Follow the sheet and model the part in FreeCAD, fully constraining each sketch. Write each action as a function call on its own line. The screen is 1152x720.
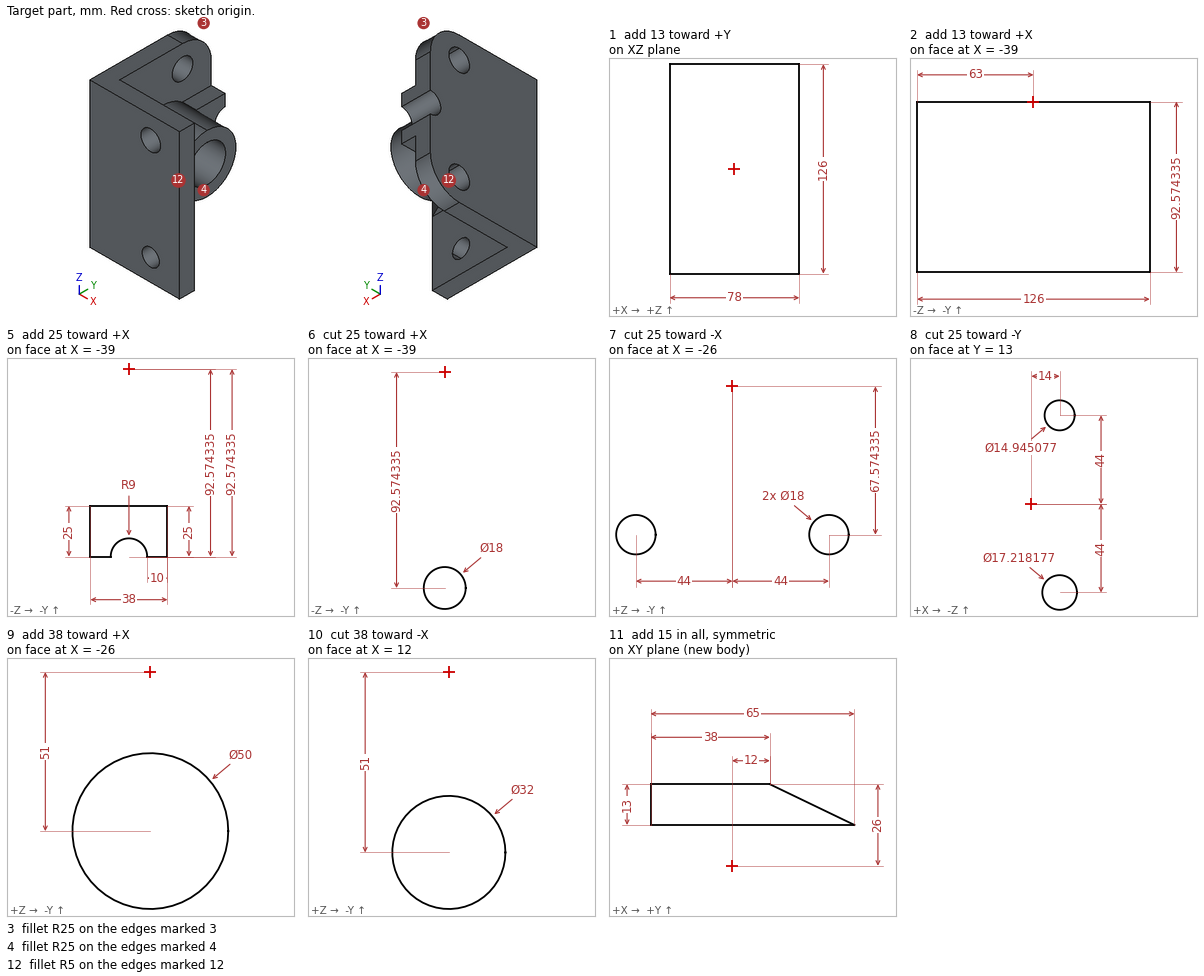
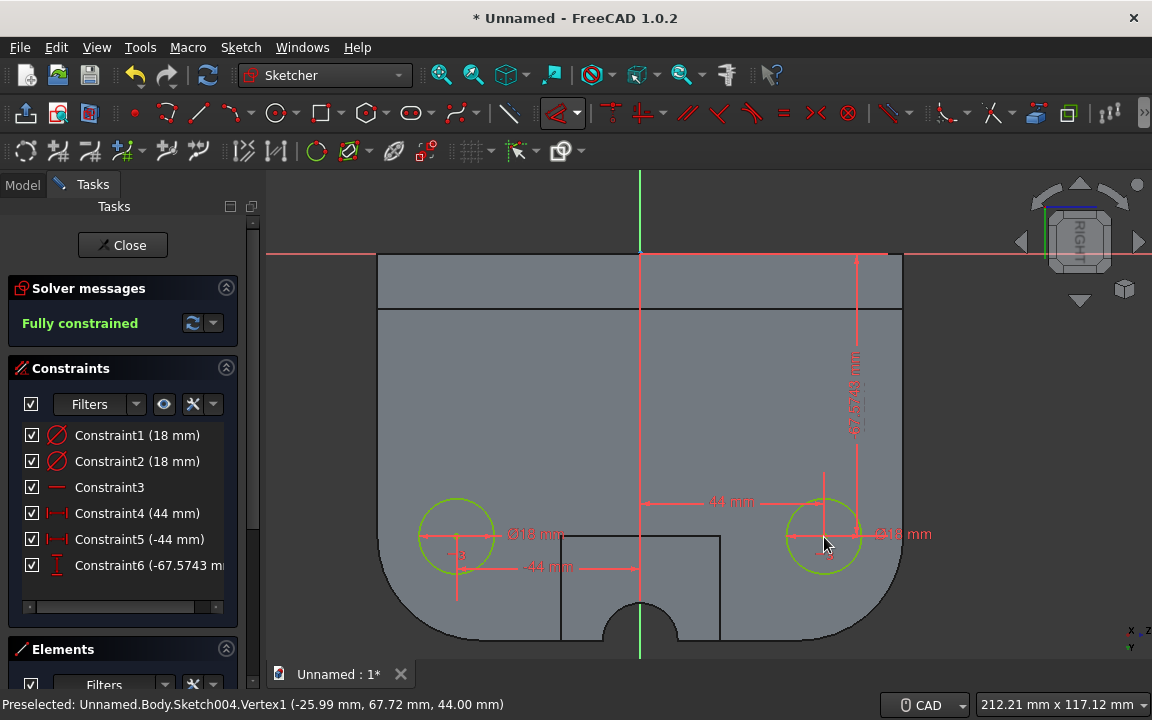
click(123, 245)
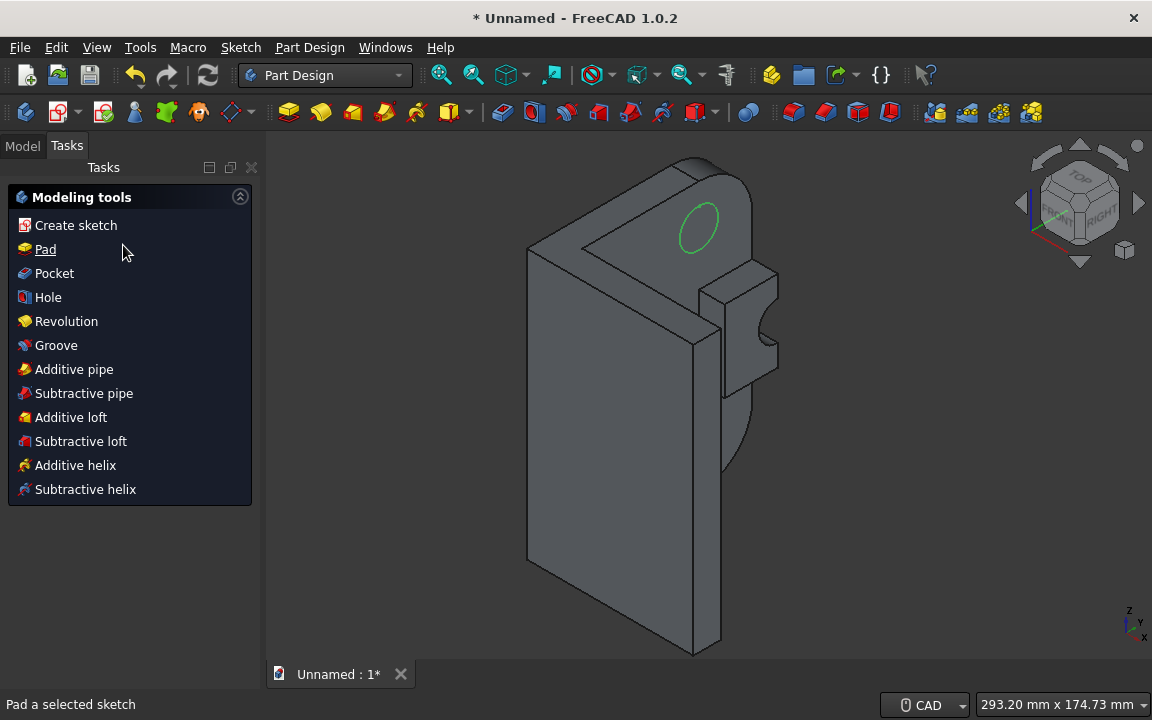
click(504, 112)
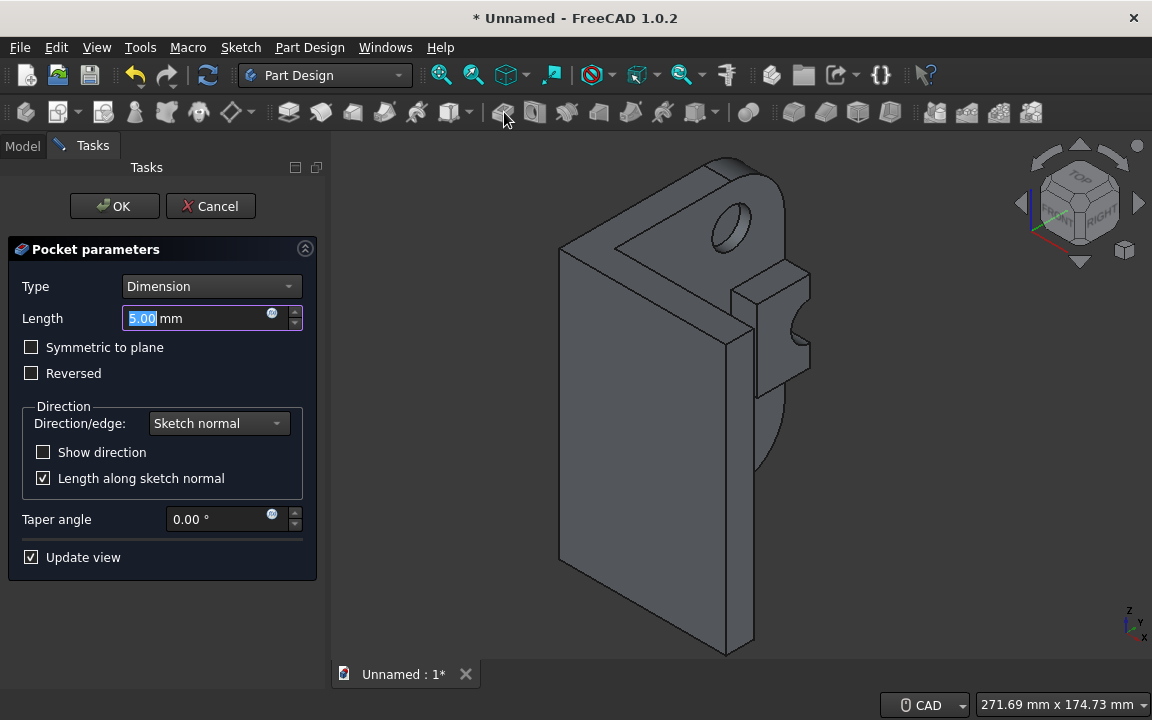
text(25)
key(Tab)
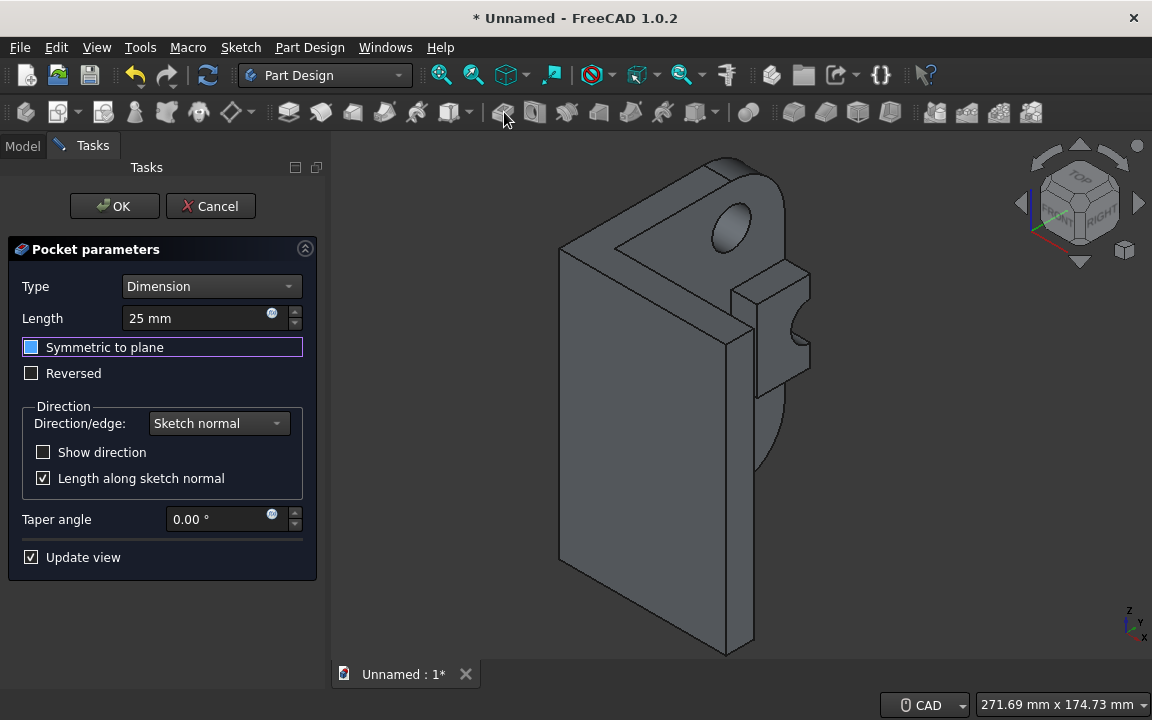
click(115, 206)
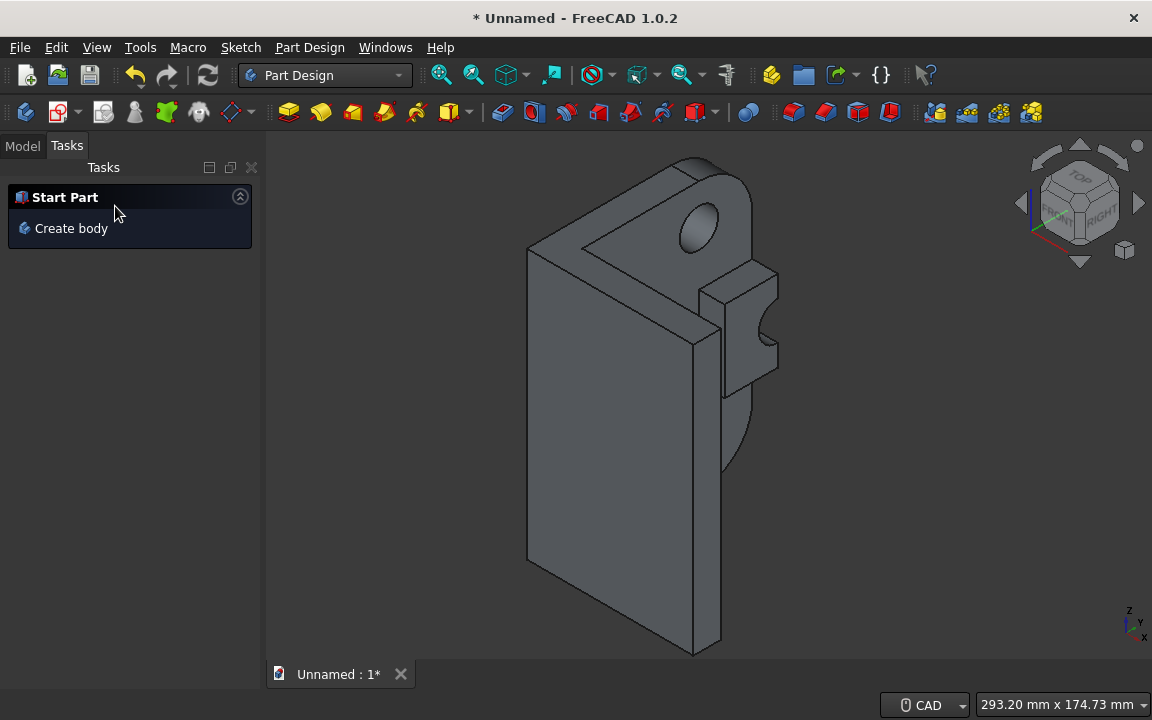
key(4)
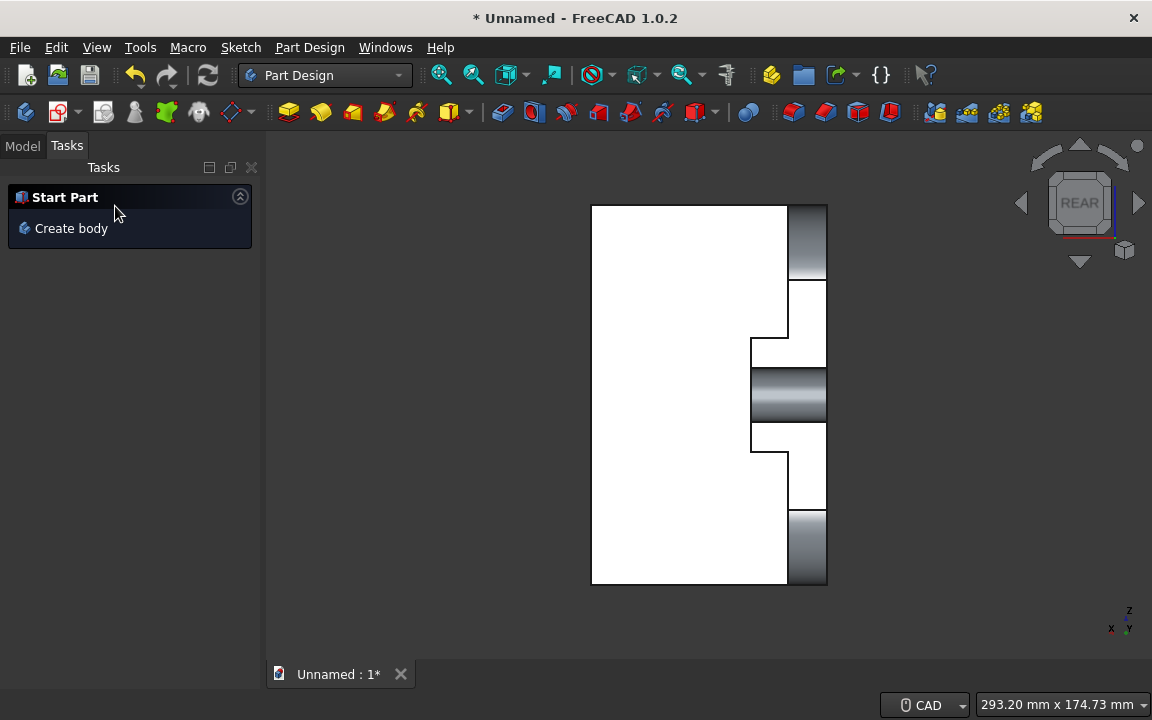
click(689, 340)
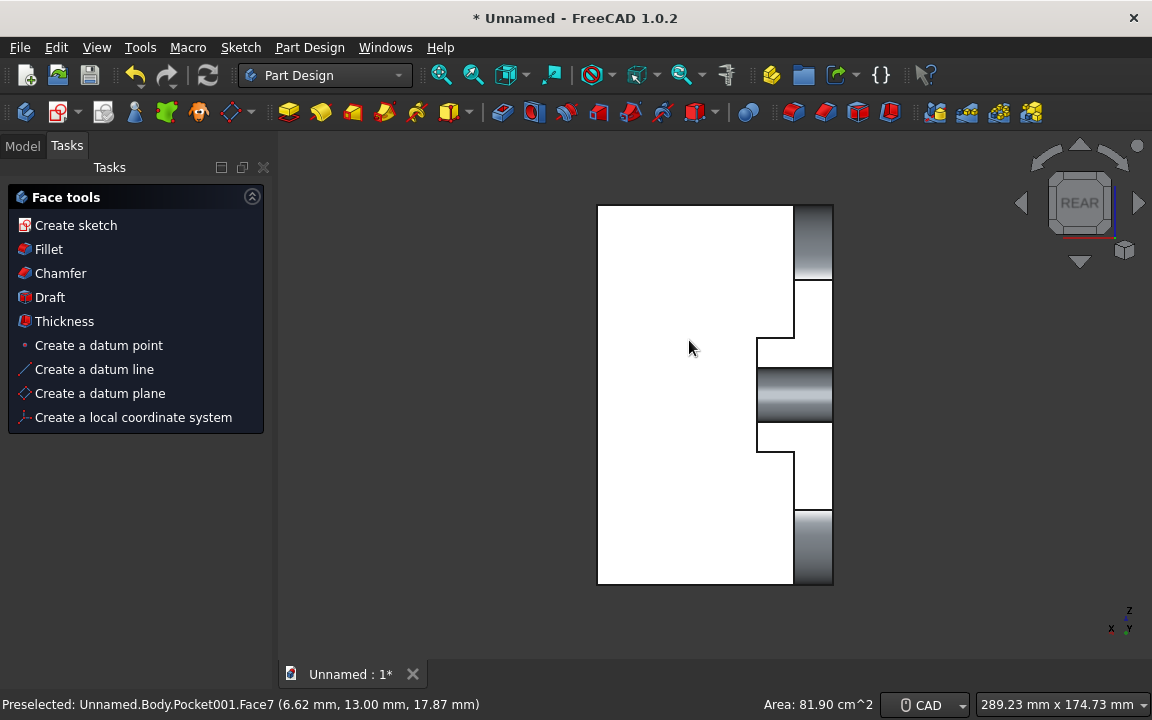
click(58, 112)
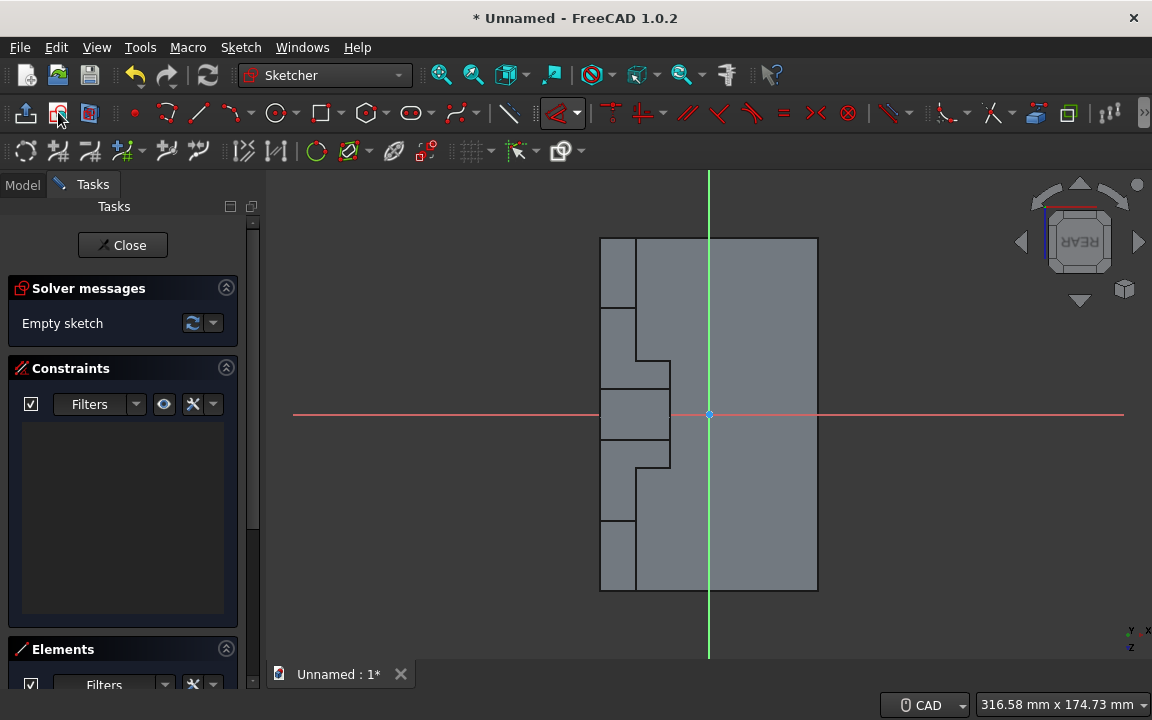
key(q)
key(s)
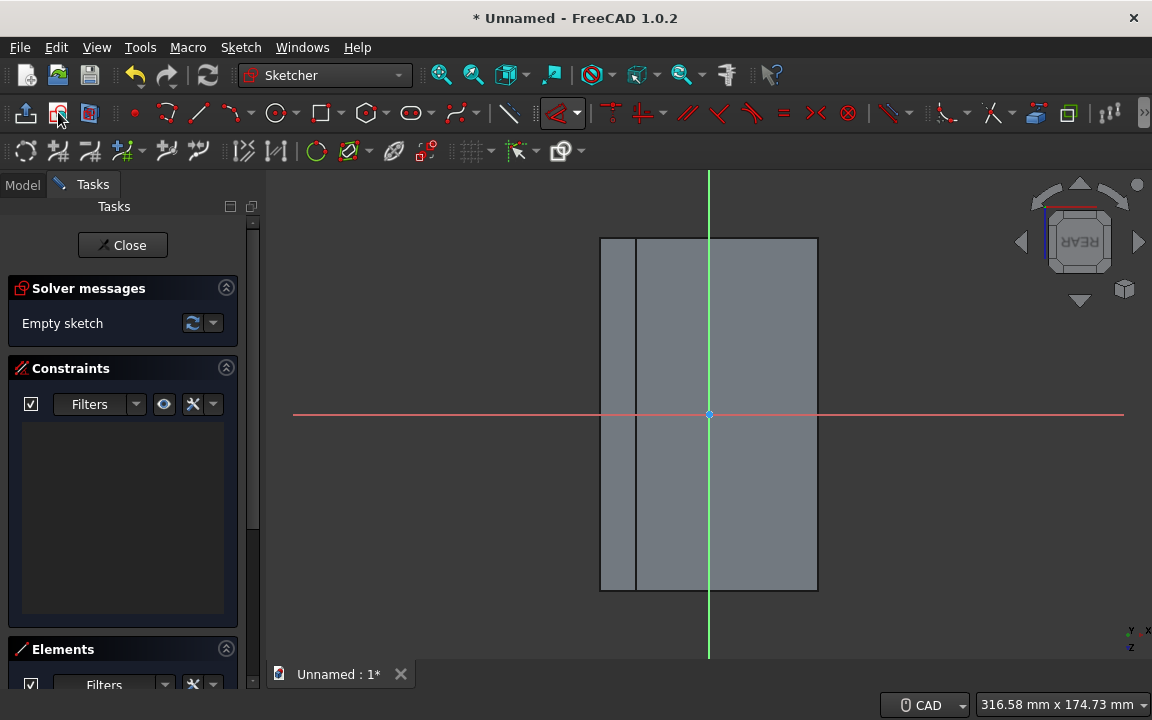
click(276, 114)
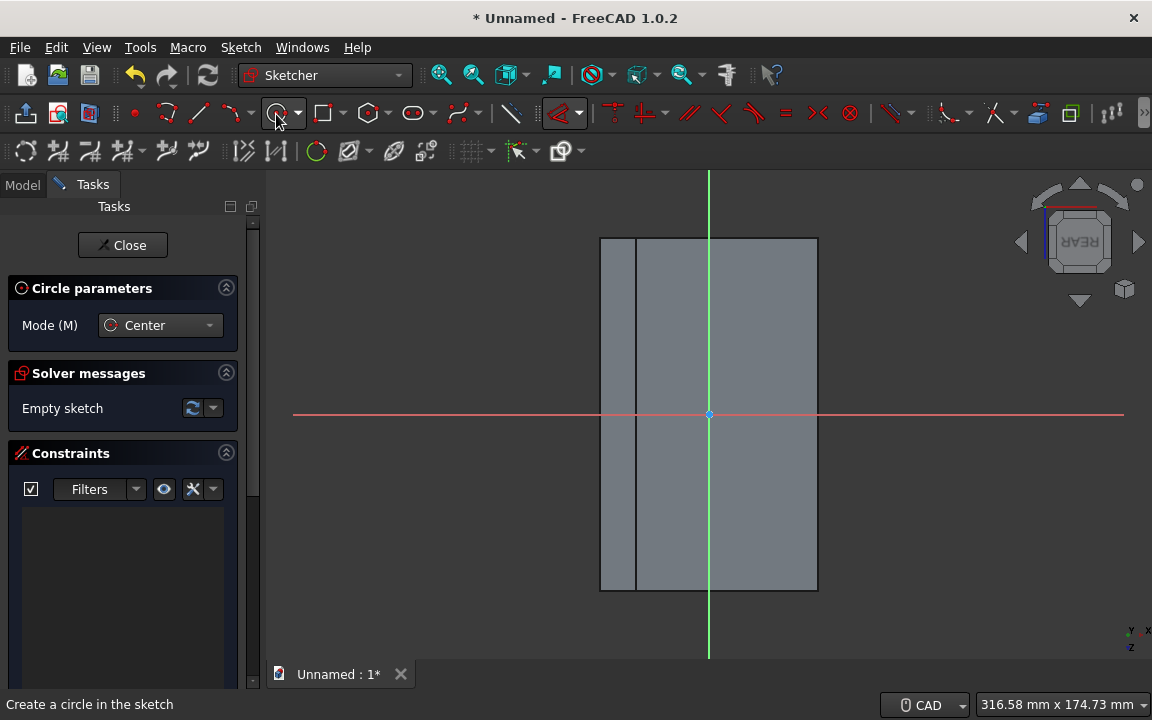
click(748, 291)
move(763, 277)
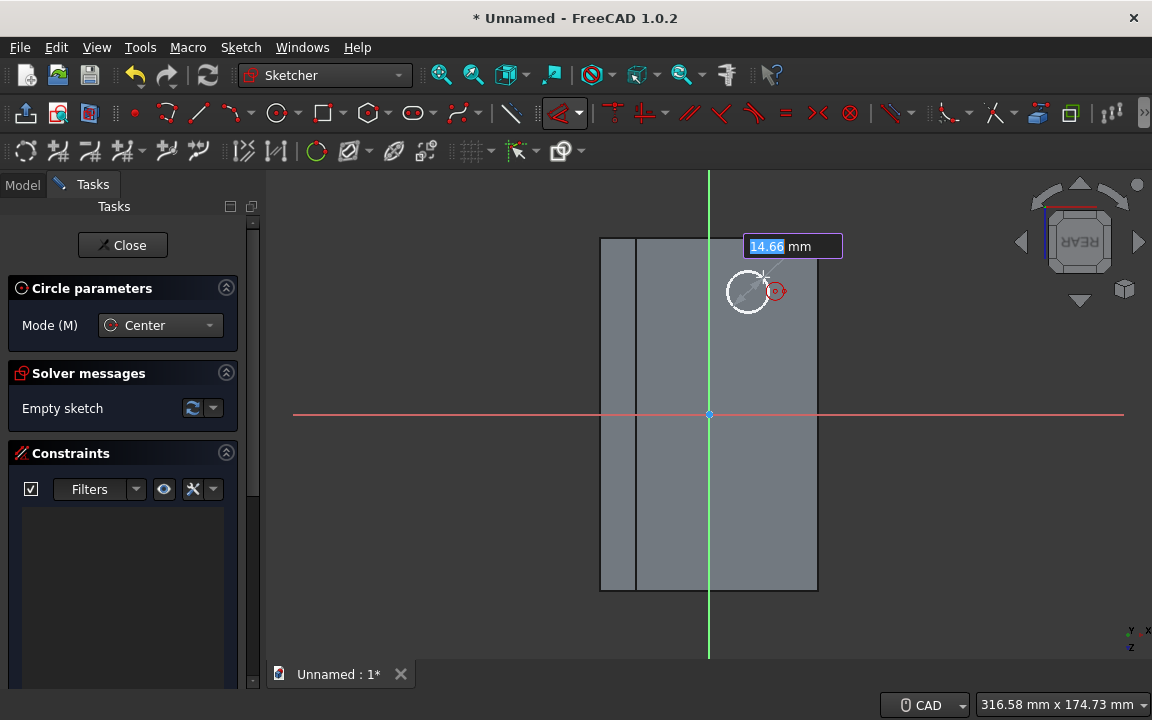
text(14.945077)
key(Return)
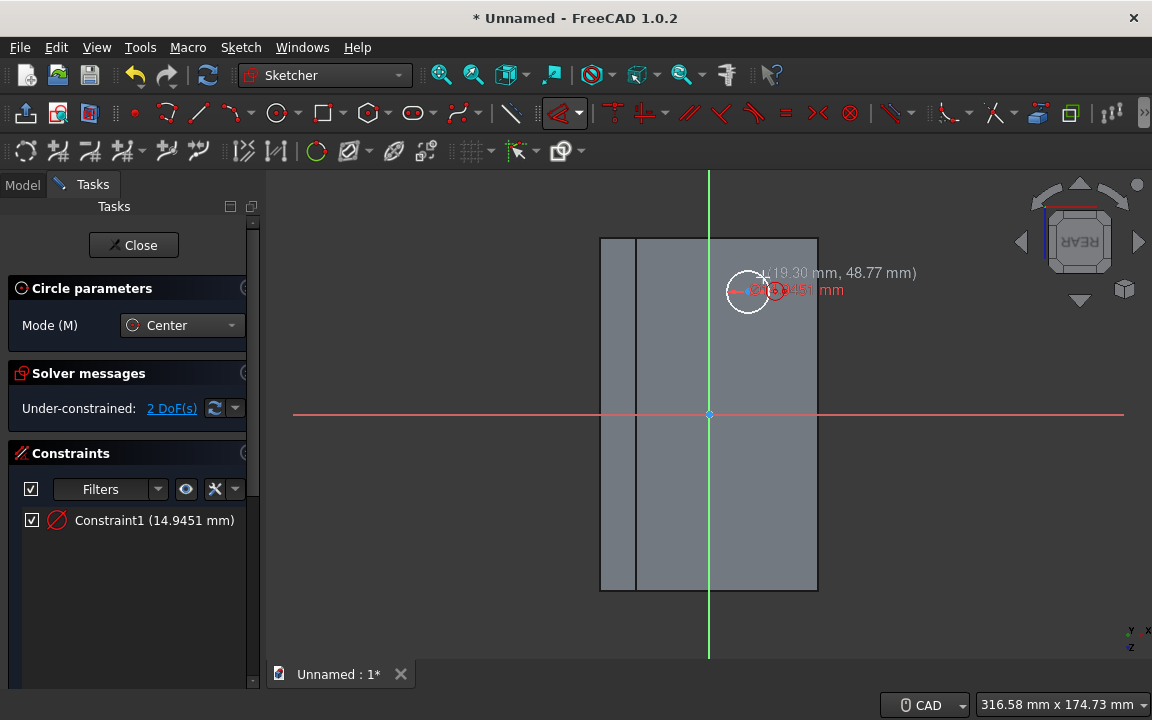
click(748, 538)
move(765, 521)